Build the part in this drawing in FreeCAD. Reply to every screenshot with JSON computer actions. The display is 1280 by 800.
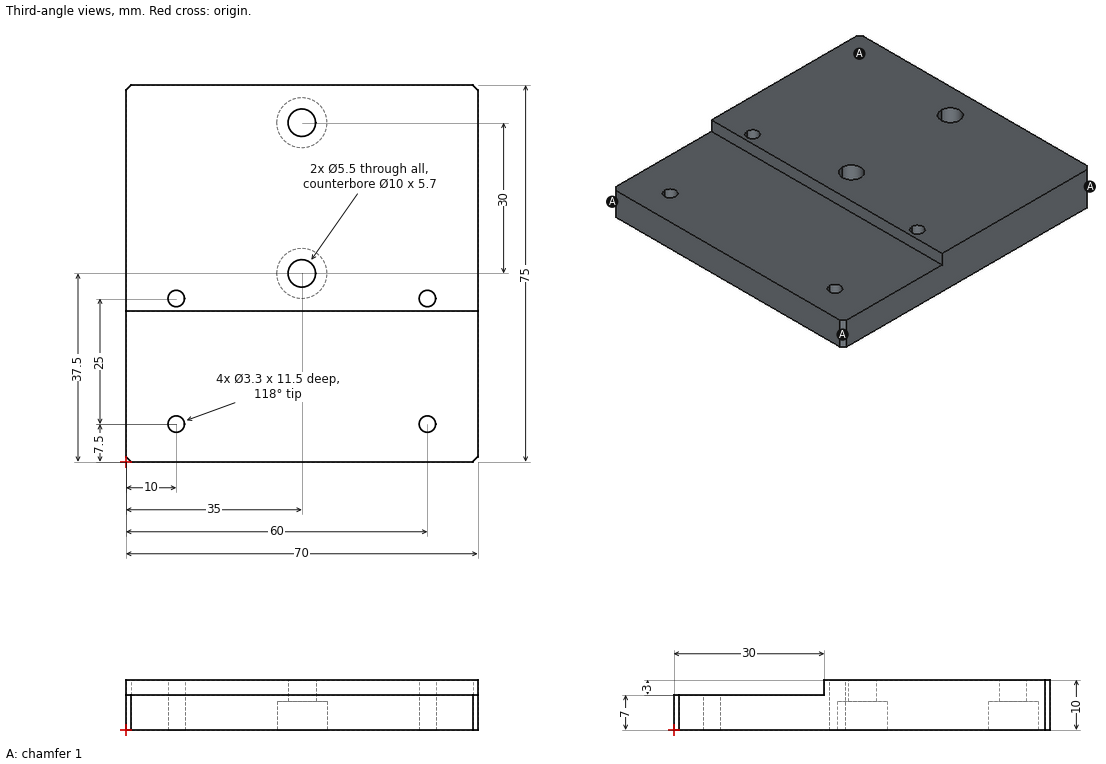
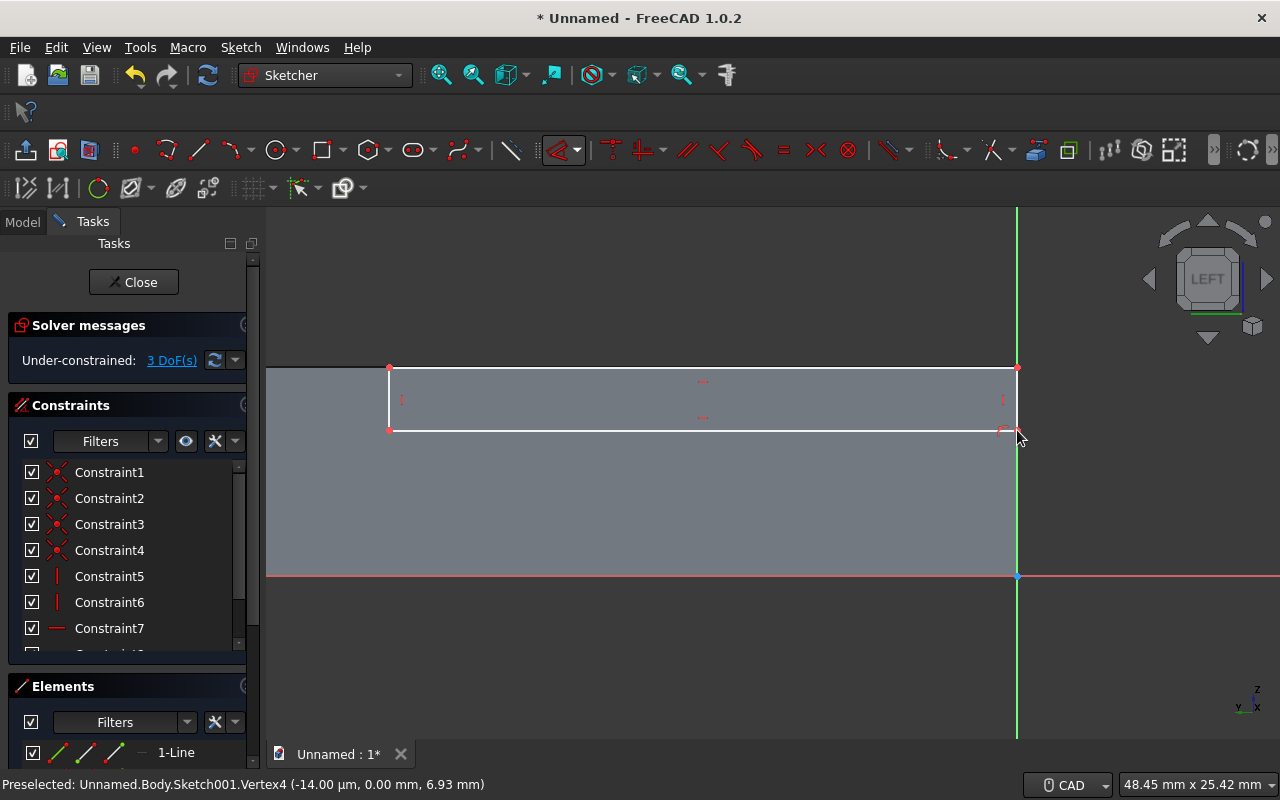
{"action": "left_click", "coordinate": [558, 150]}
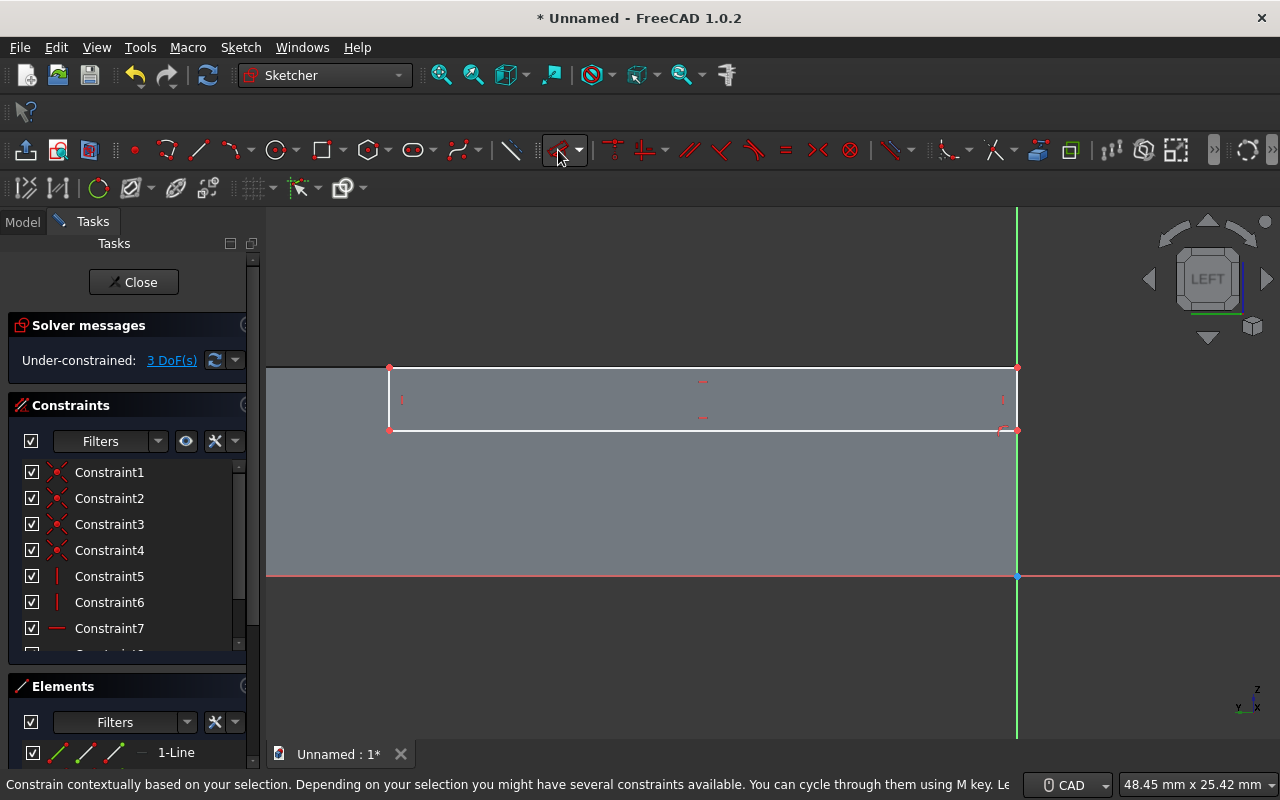
{"action": "left_click", "coordinate": [389, 387]}
{"action": "left_click", "coordinate": [355, 399]}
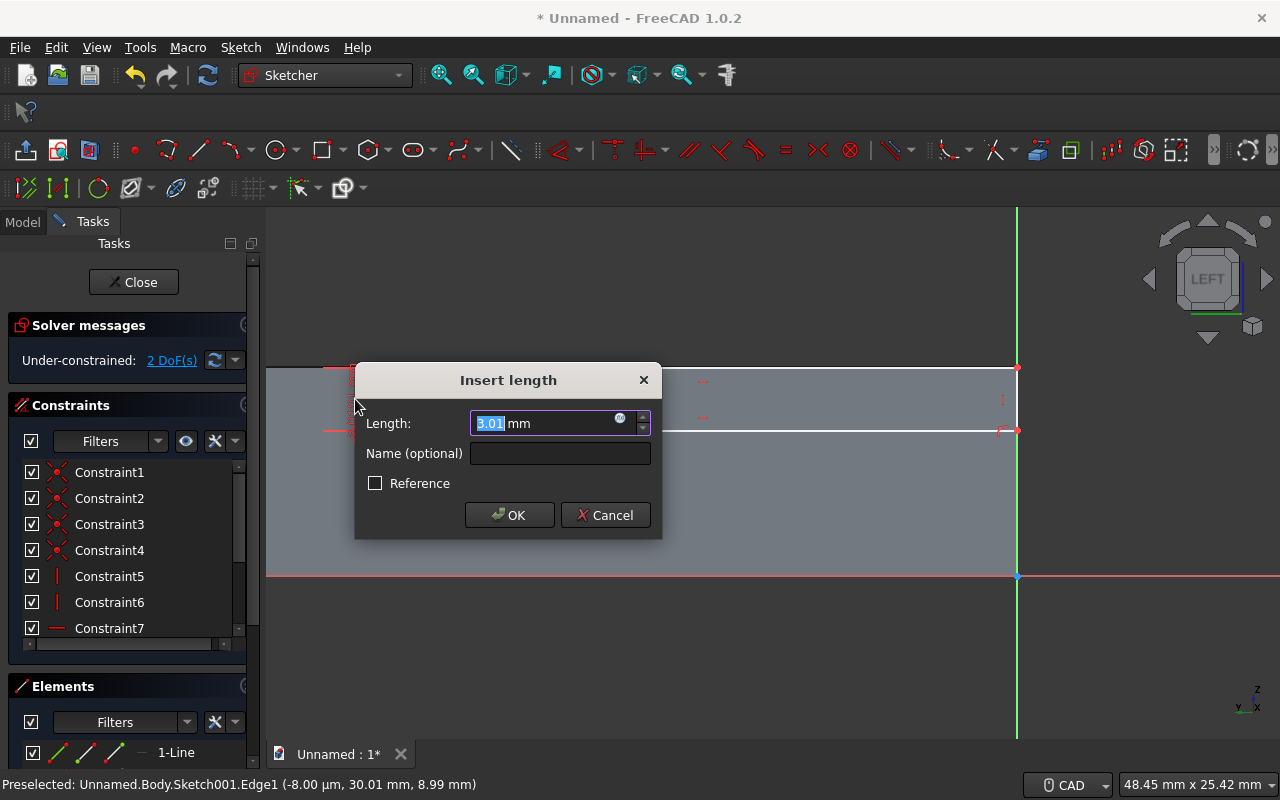
{"action": "type", "text": "3"}
{"action": "key", "text": "Return"}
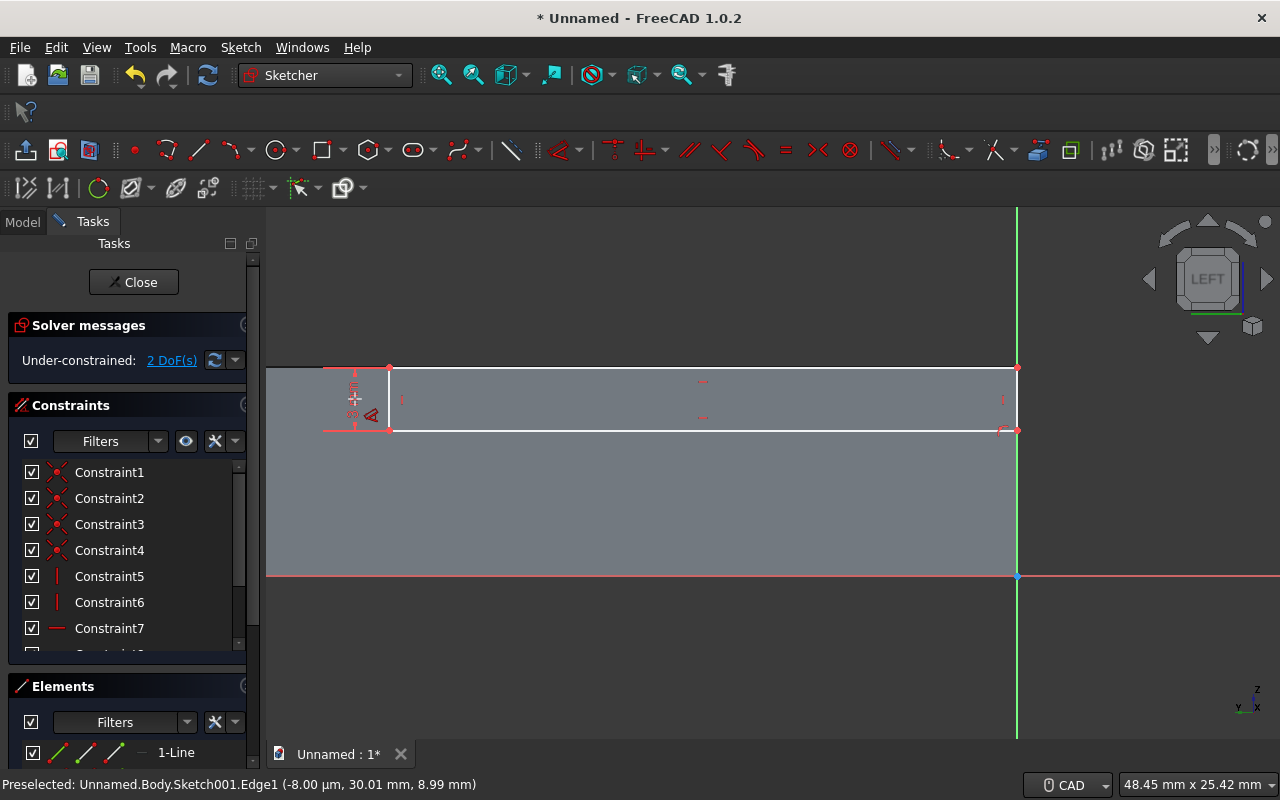
{"action": "left_click", "coordinate": [577, 431]}
{"action": "left_click", "coordinate": [703, 397]}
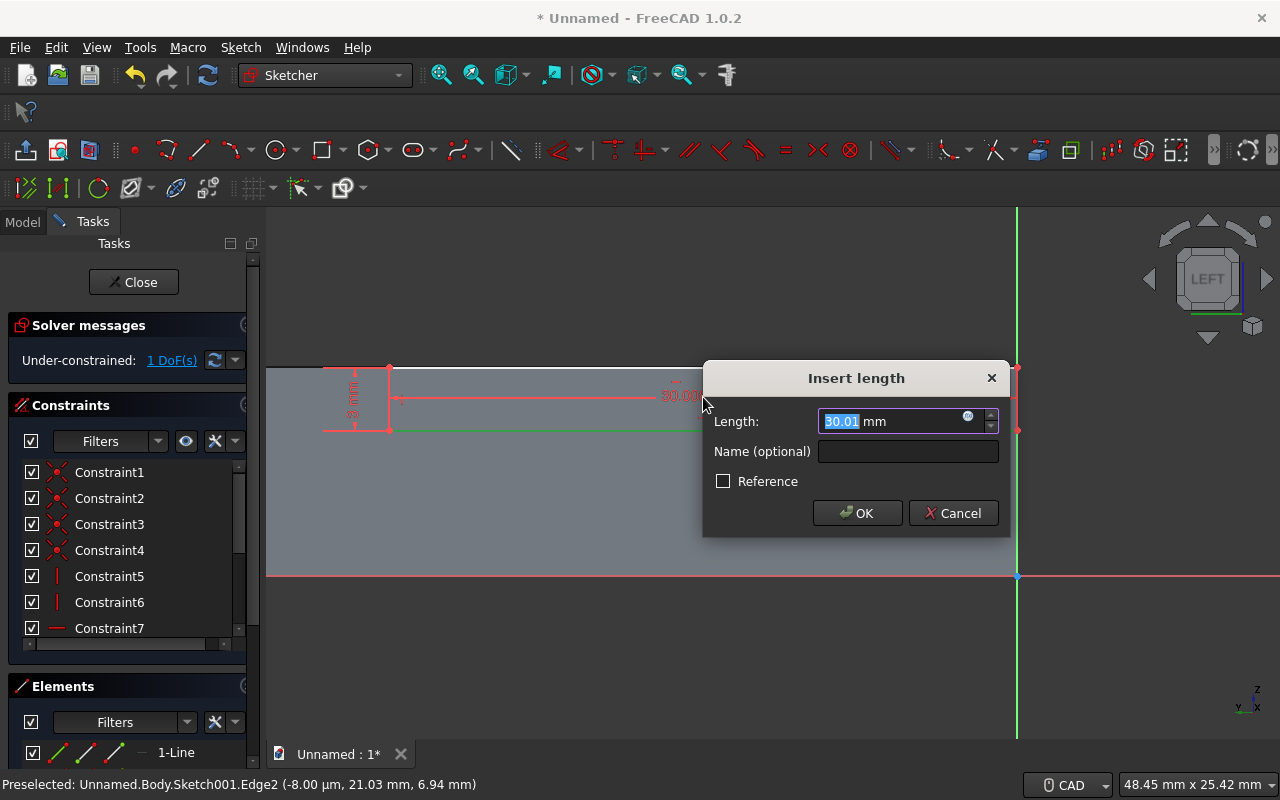
{"action": "type", "text": "30"}
{"action": "key", "text": "Return"}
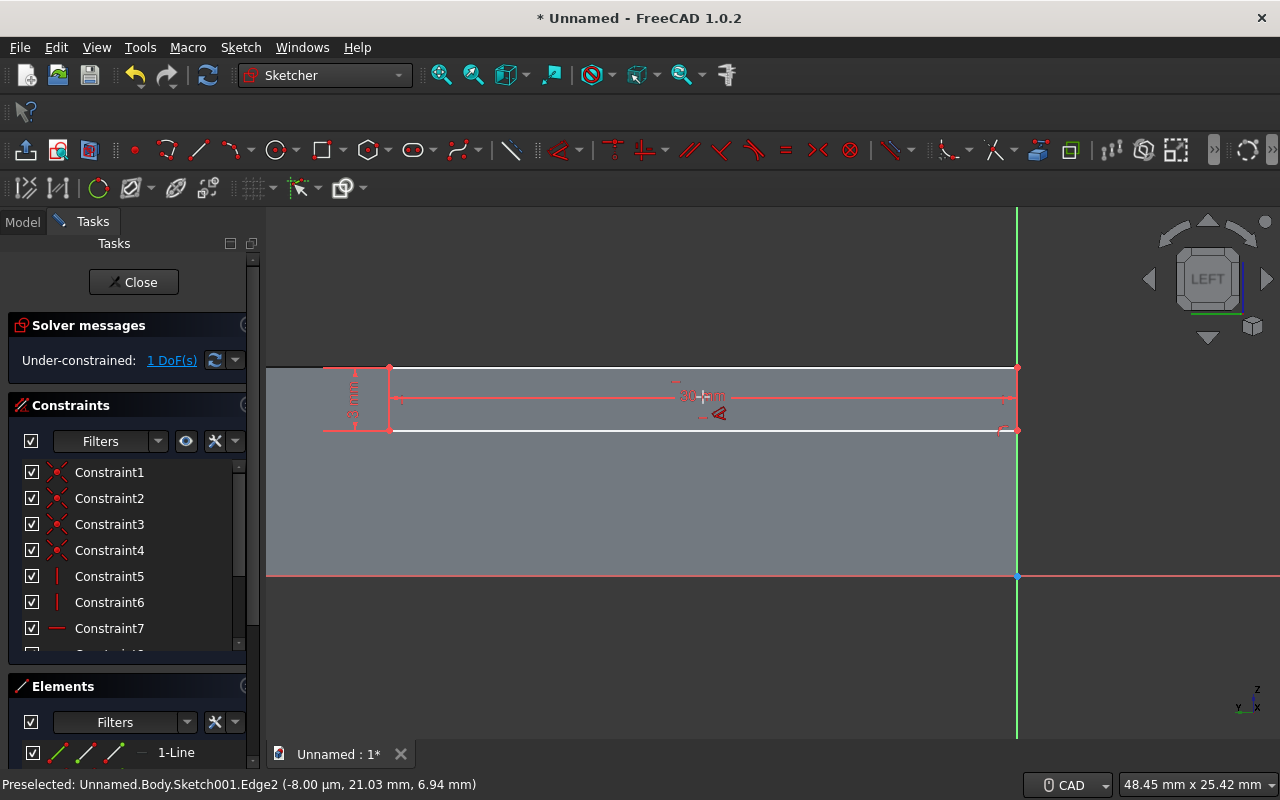
{"action": "left_click", "coordinate": [389, 431]}
{"action": "left_click", "coordinate": [1051, 503]}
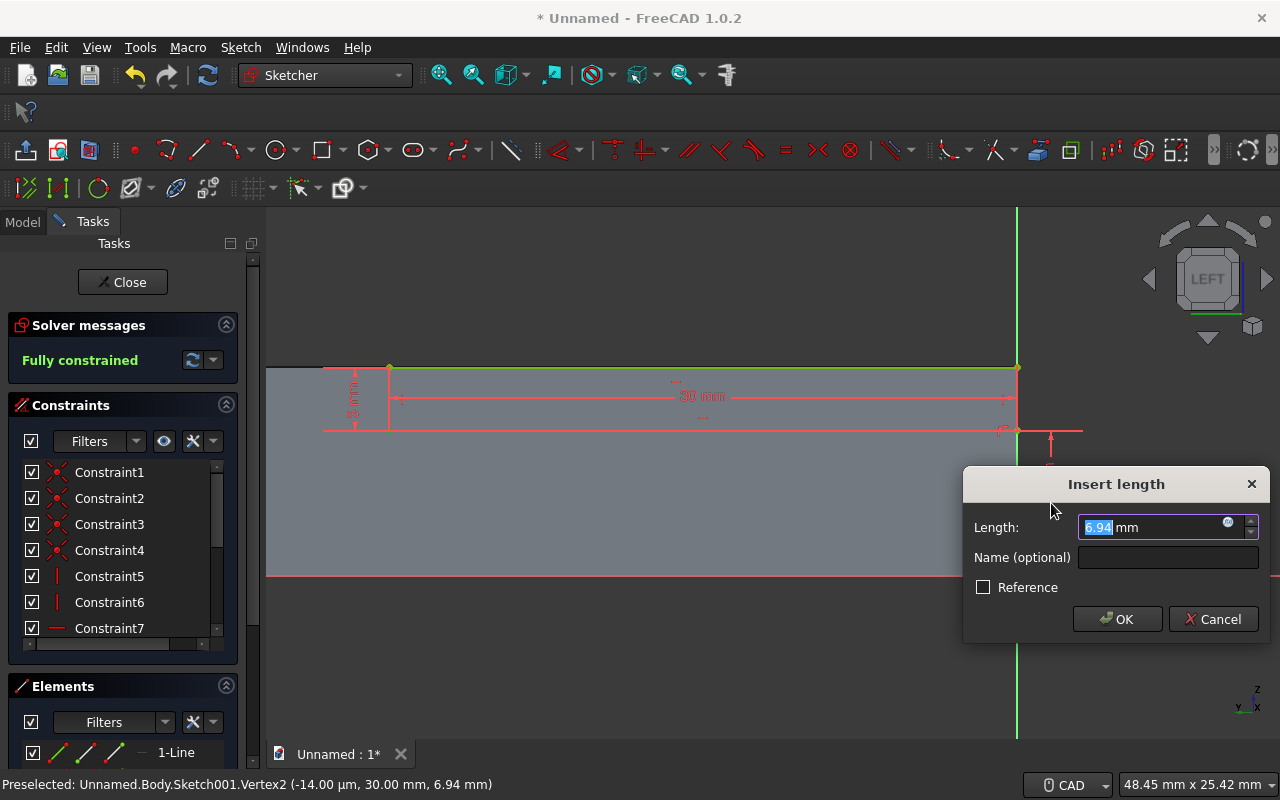
{"action": "type", "text": "7"}
{"action": "key", "text": "Return"}
{"action": "key", "text": "Escape"}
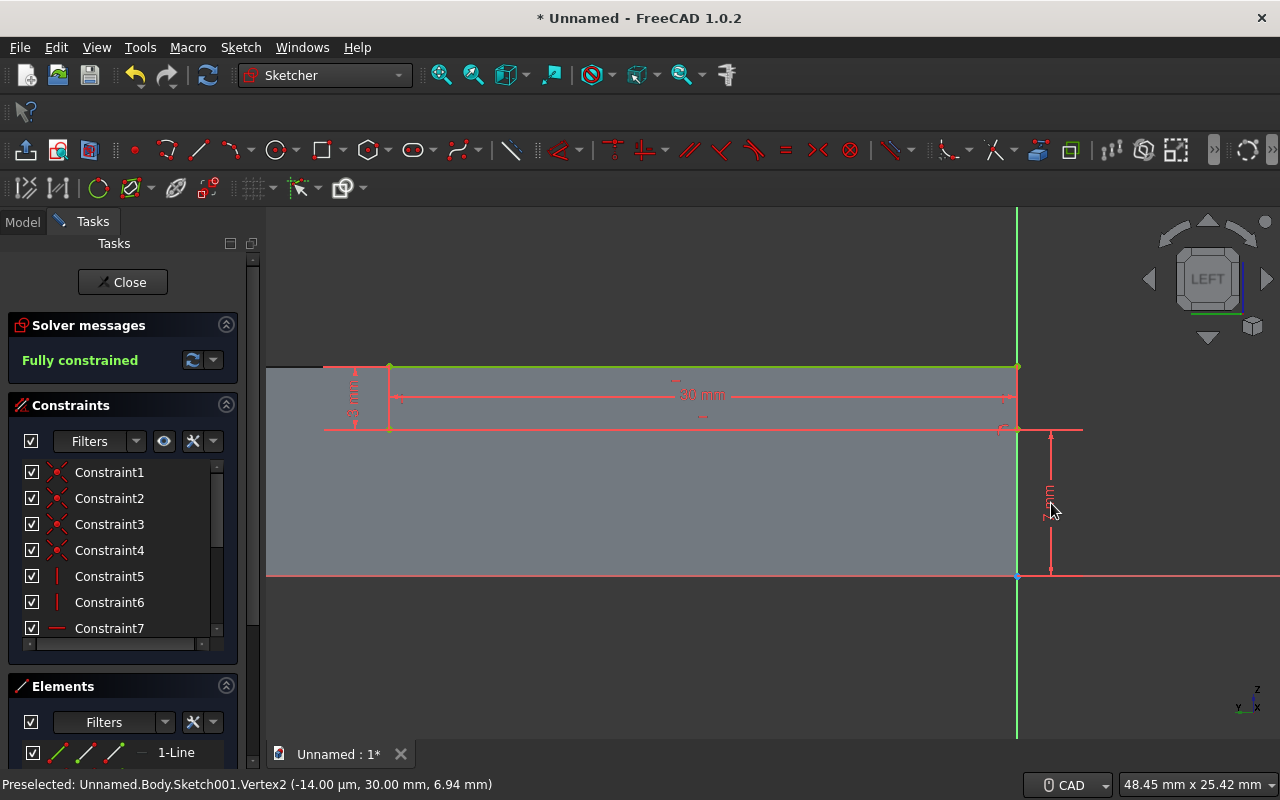
{"action": "left_click", "coordinate": [123, 282]}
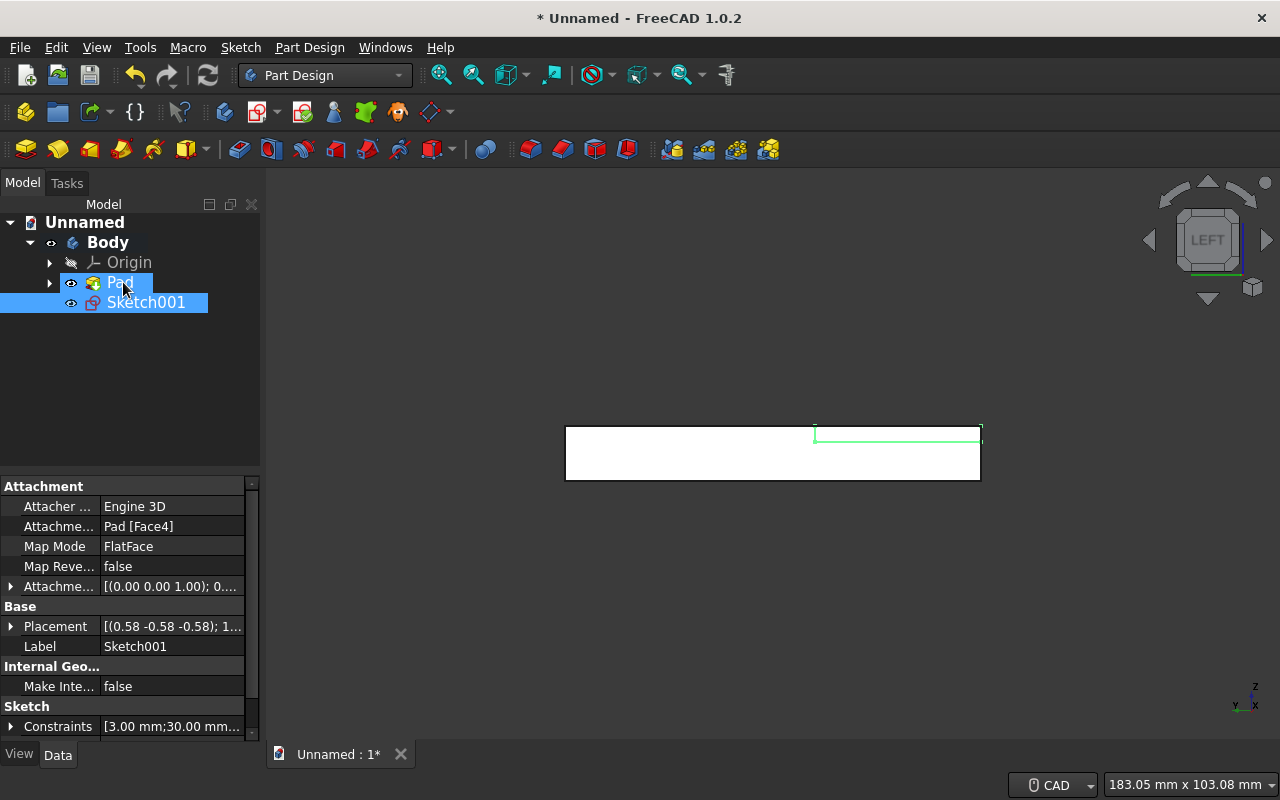
{"action": "left_click", "coordinate": [240, 150]}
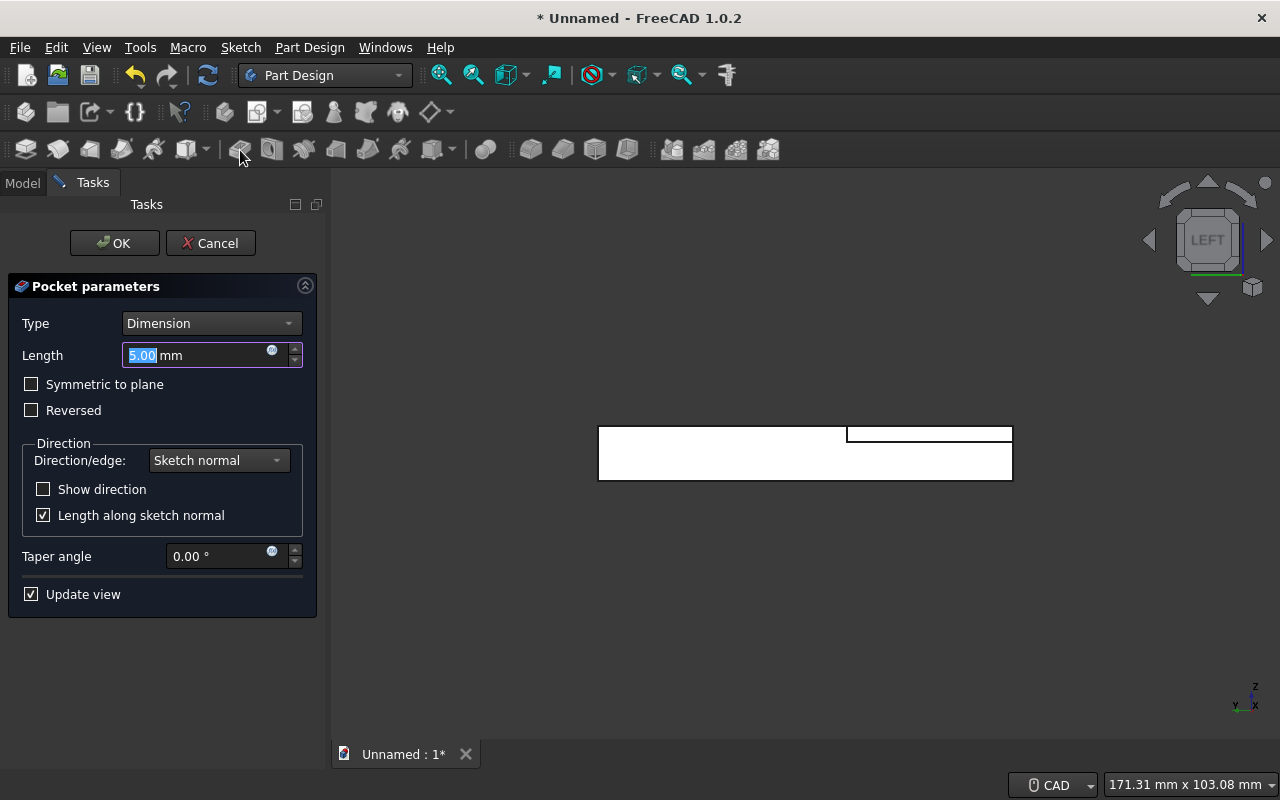
{"action": "left_click", "coordinate": [212, 324]}